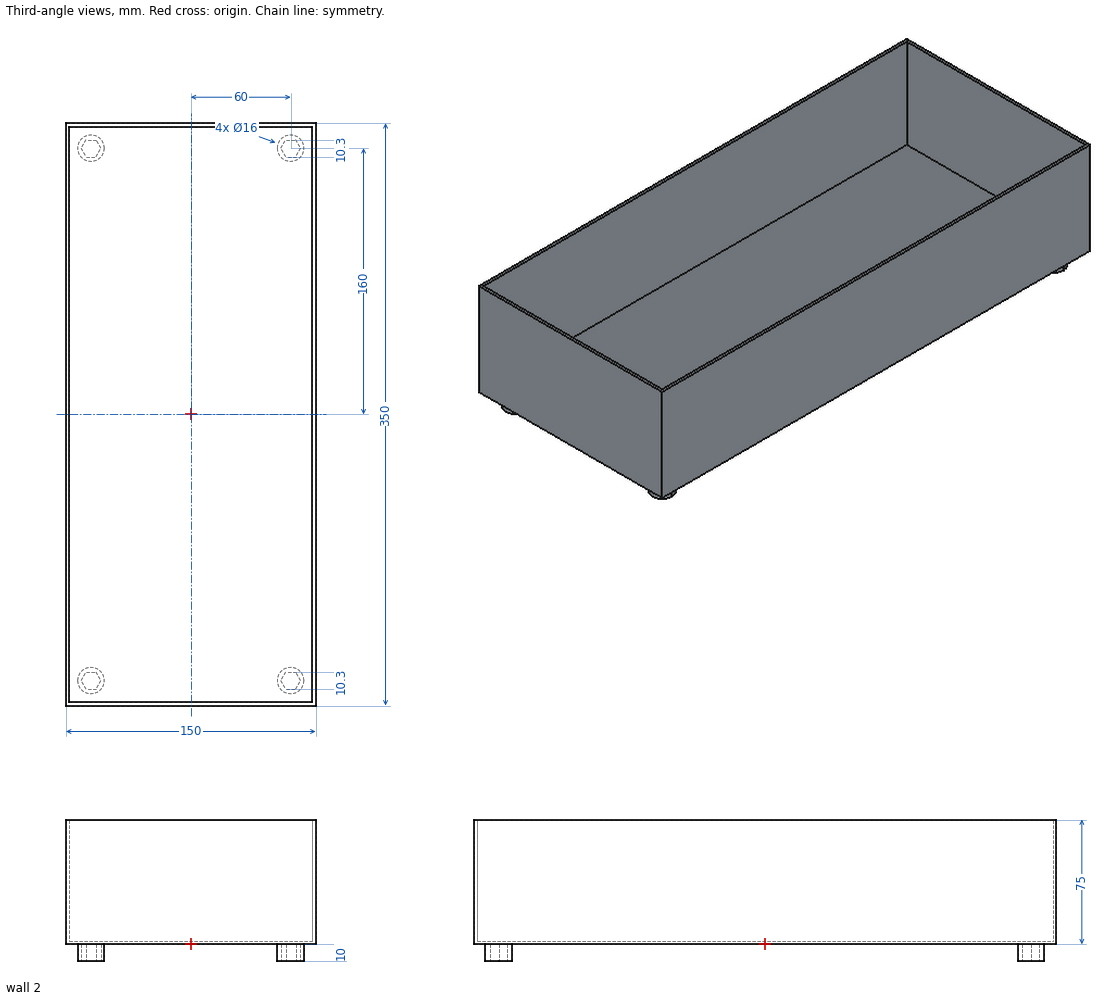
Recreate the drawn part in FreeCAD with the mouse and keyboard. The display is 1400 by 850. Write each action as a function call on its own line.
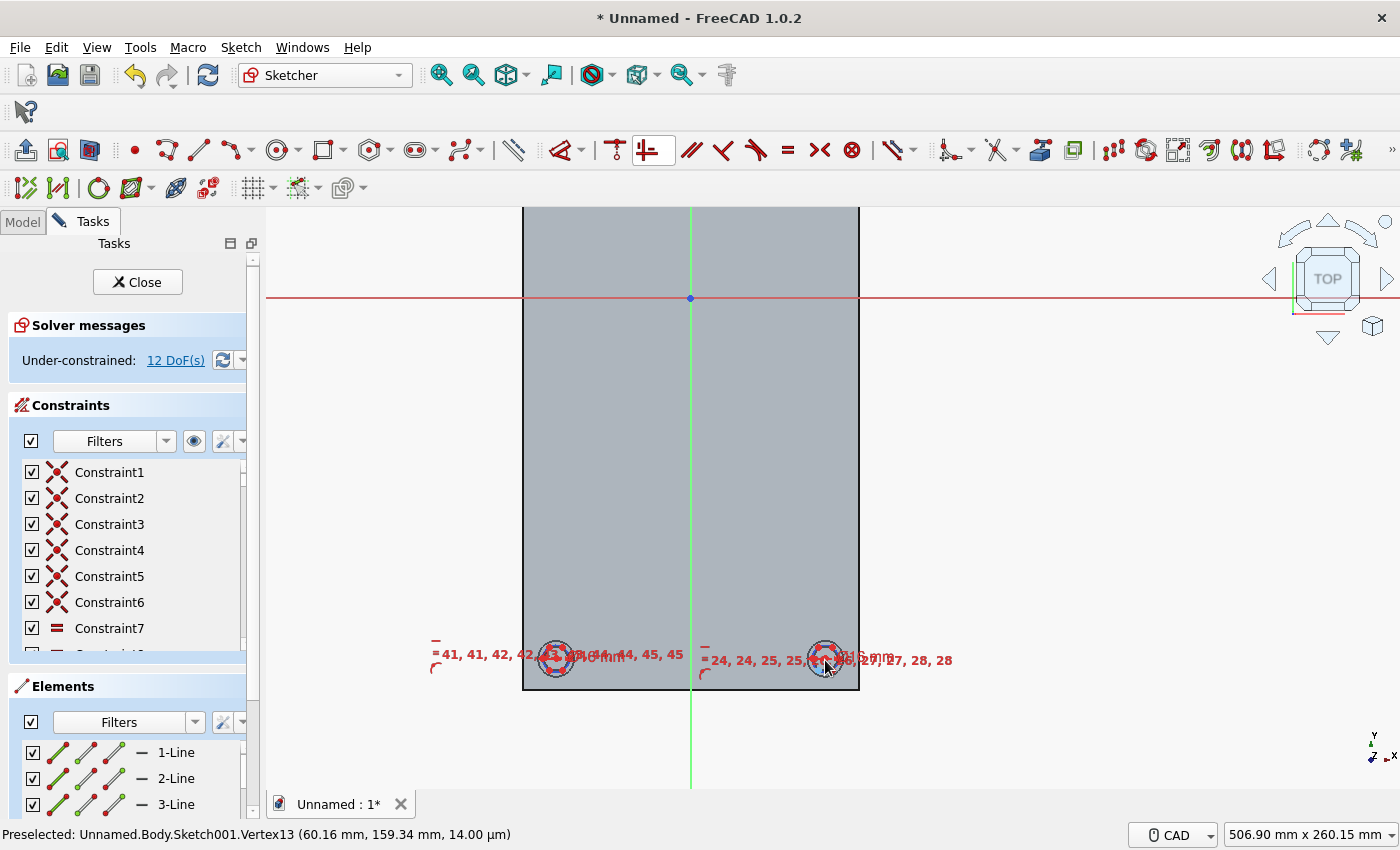
click(825, 659)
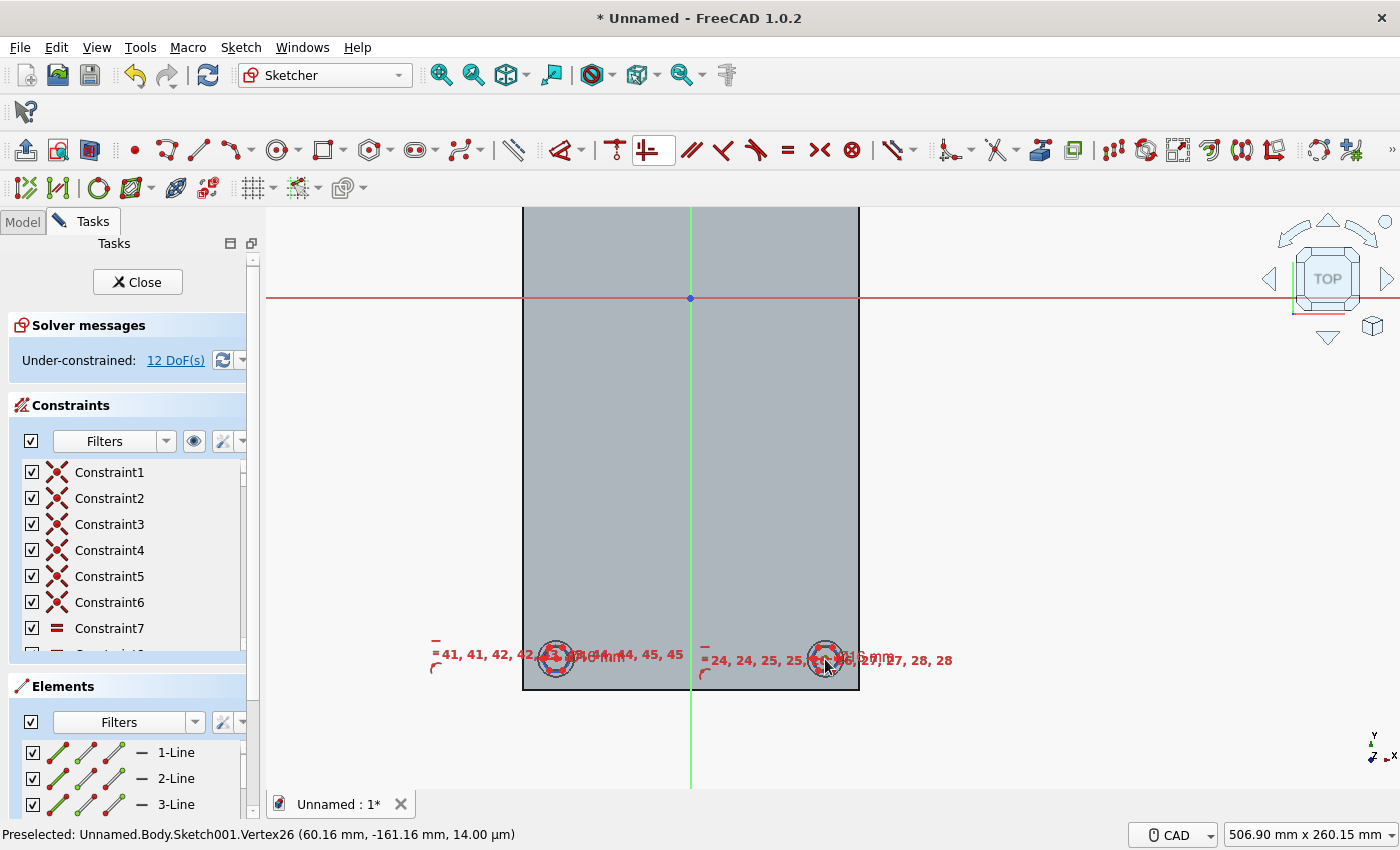
click(361, 298)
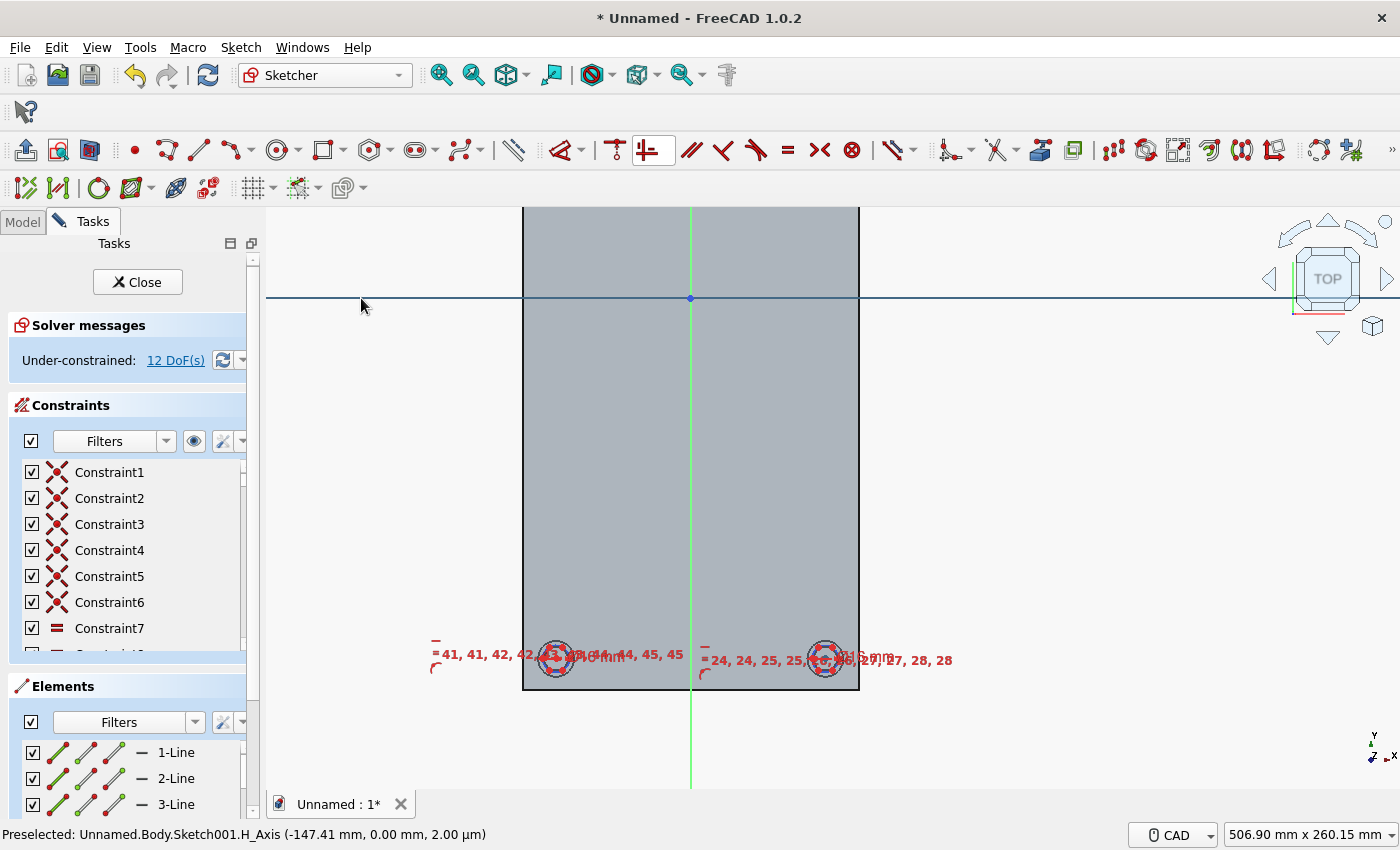
click(820, 150)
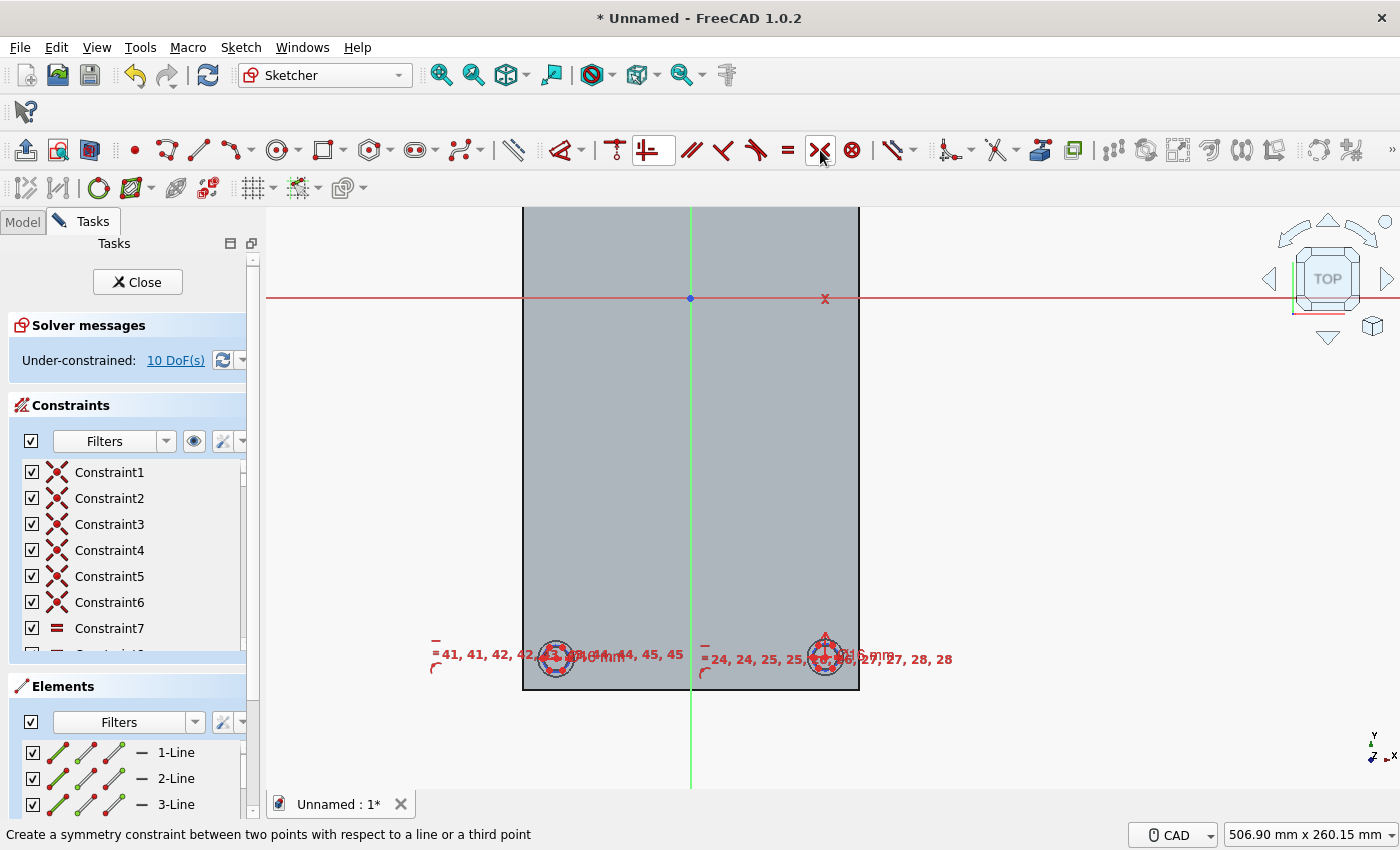
click(825, 657)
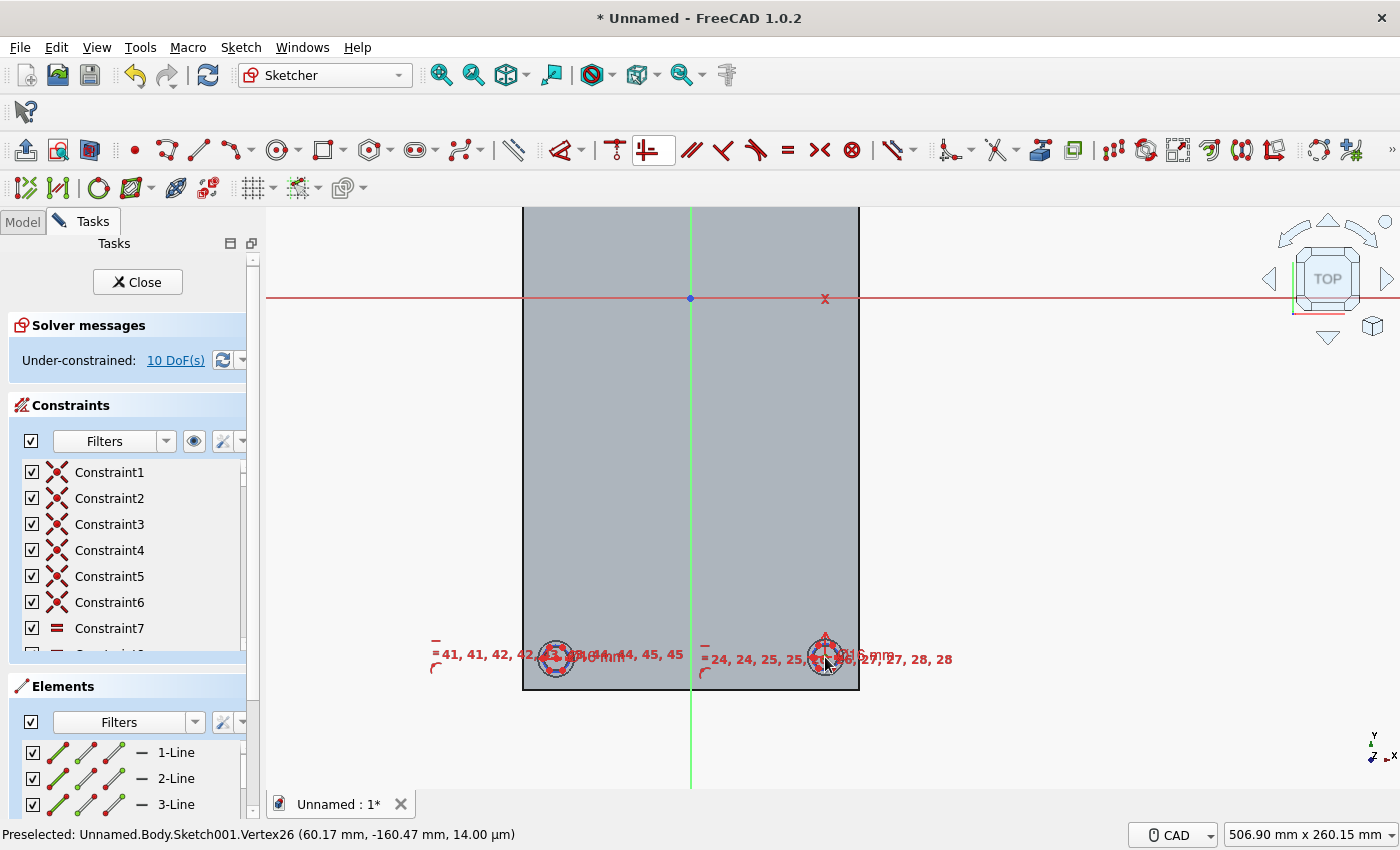
click(556, 659)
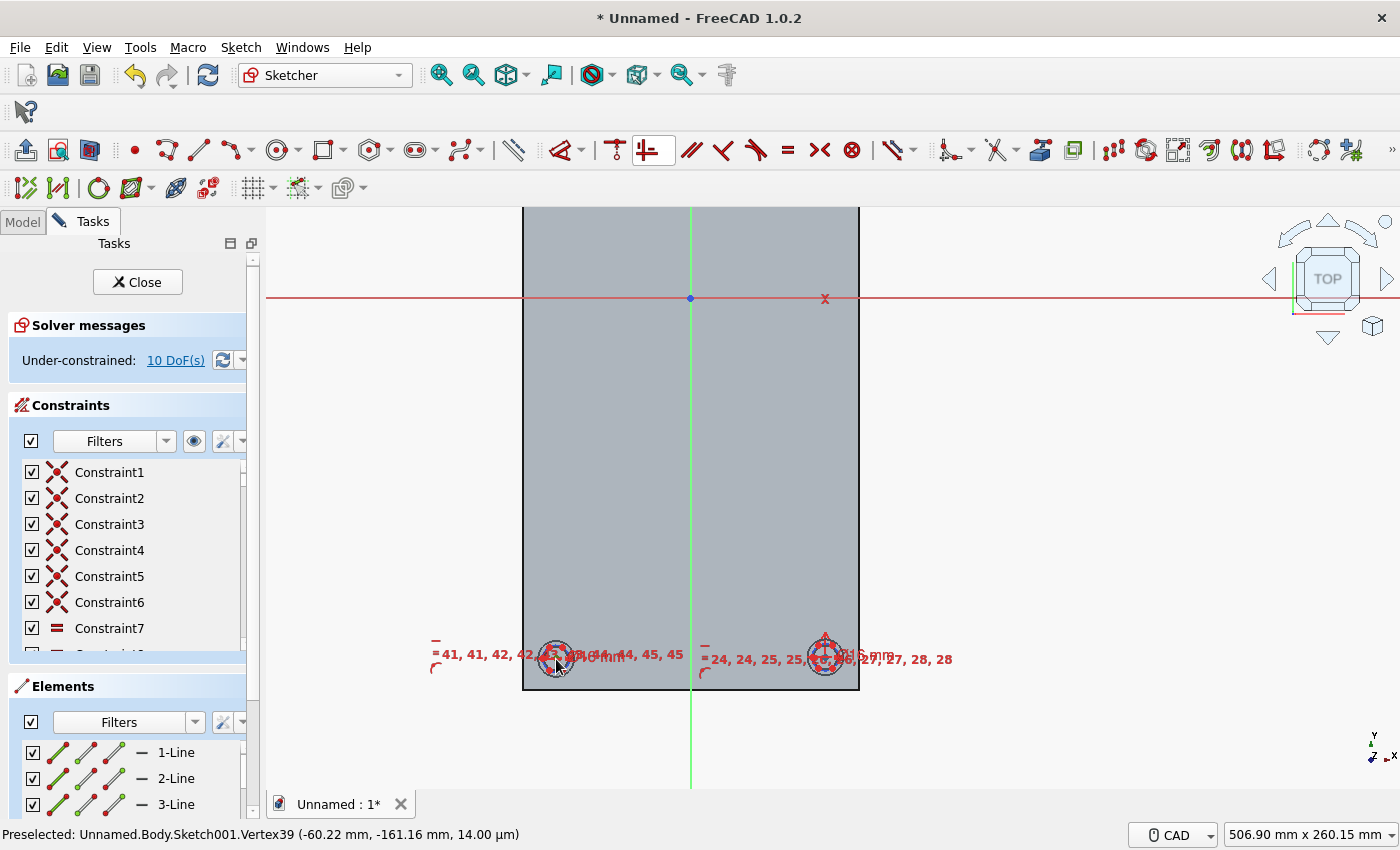
click(691, 723)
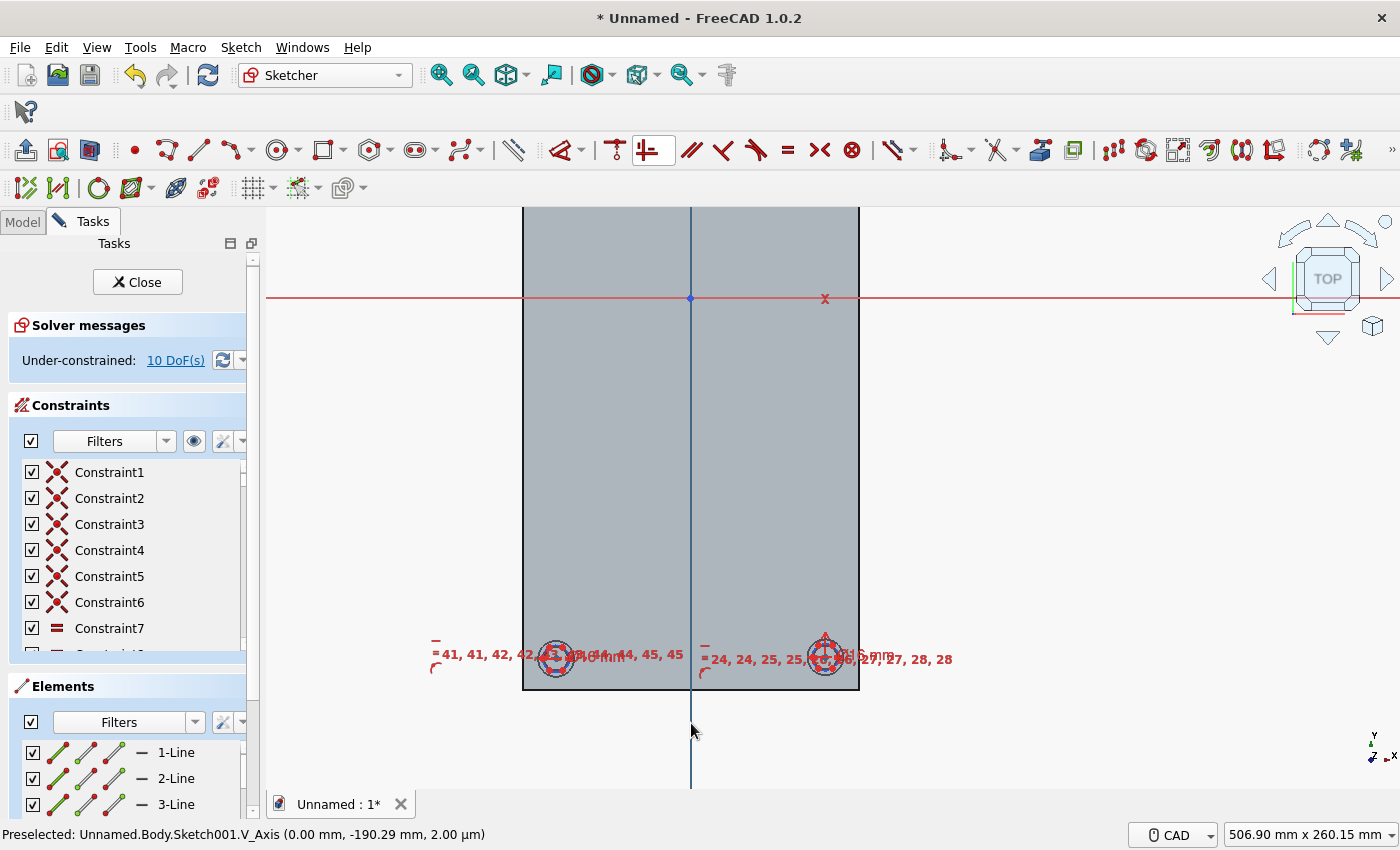
click(820, 150)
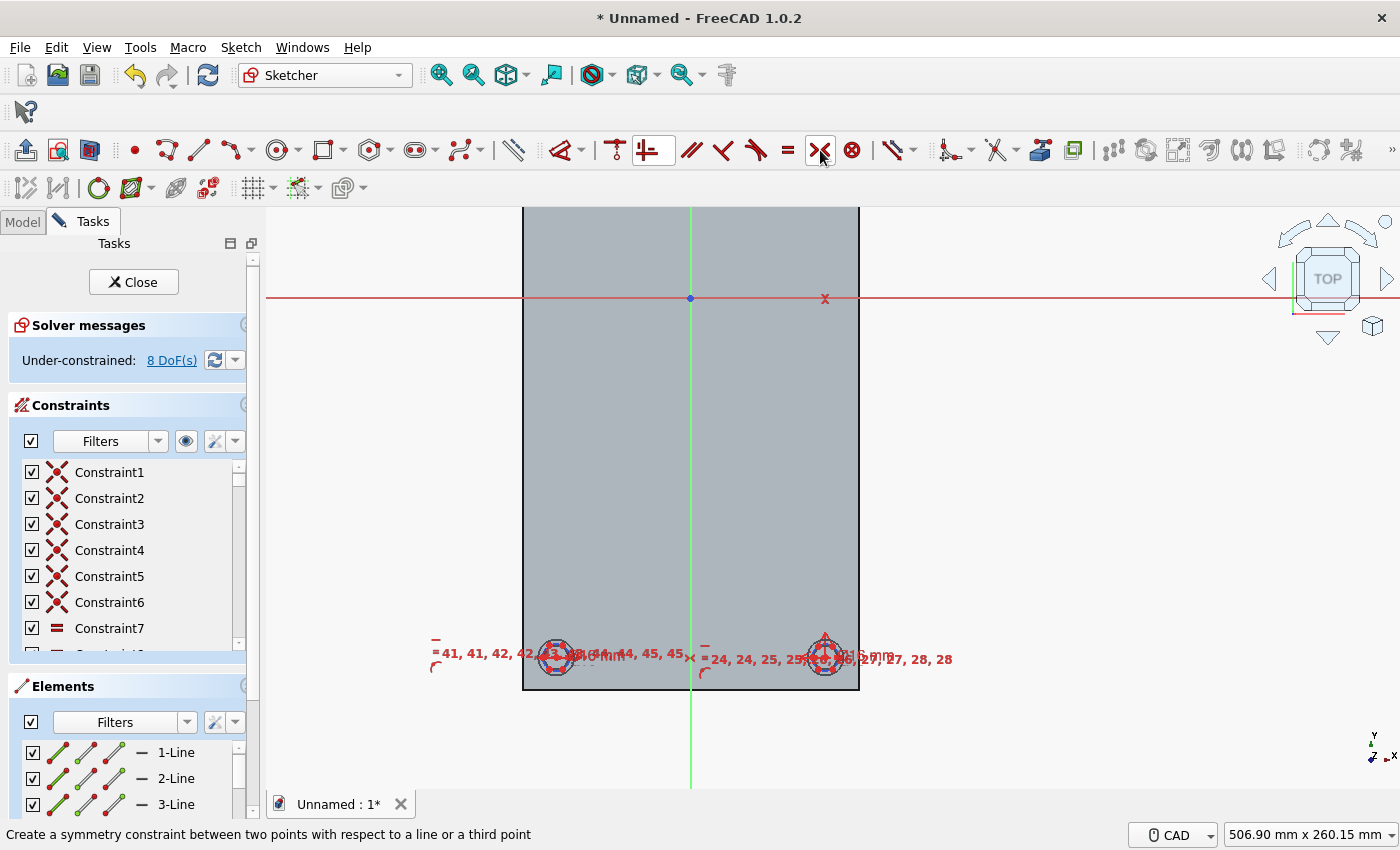
scroll(825, 661, down, 4)